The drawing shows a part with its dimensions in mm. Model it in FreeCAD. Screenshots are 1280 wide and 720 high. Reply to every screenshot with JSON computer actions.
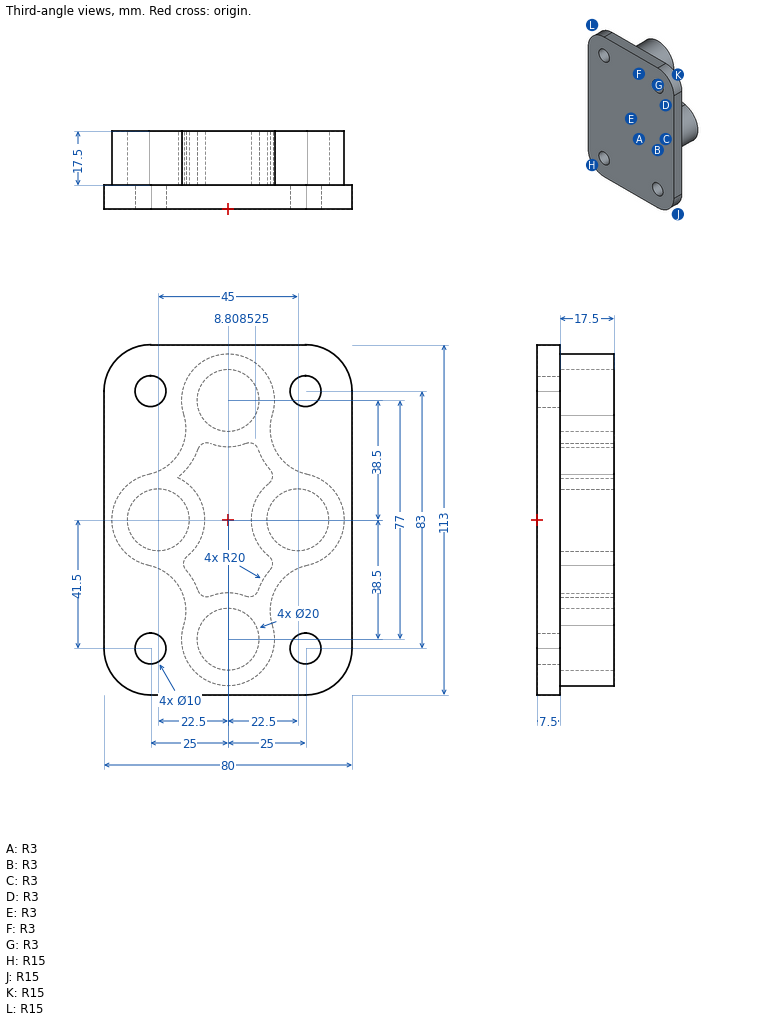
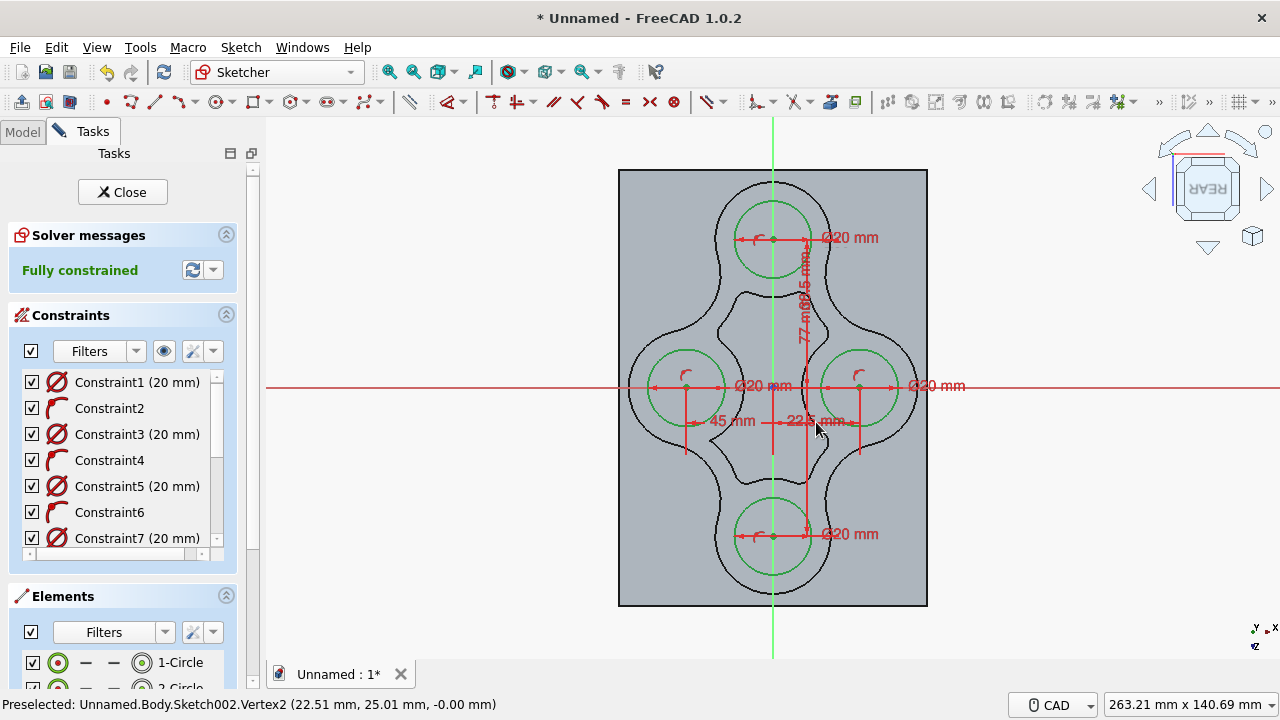
{"action": "left_click", "coordinate": [123, 192]}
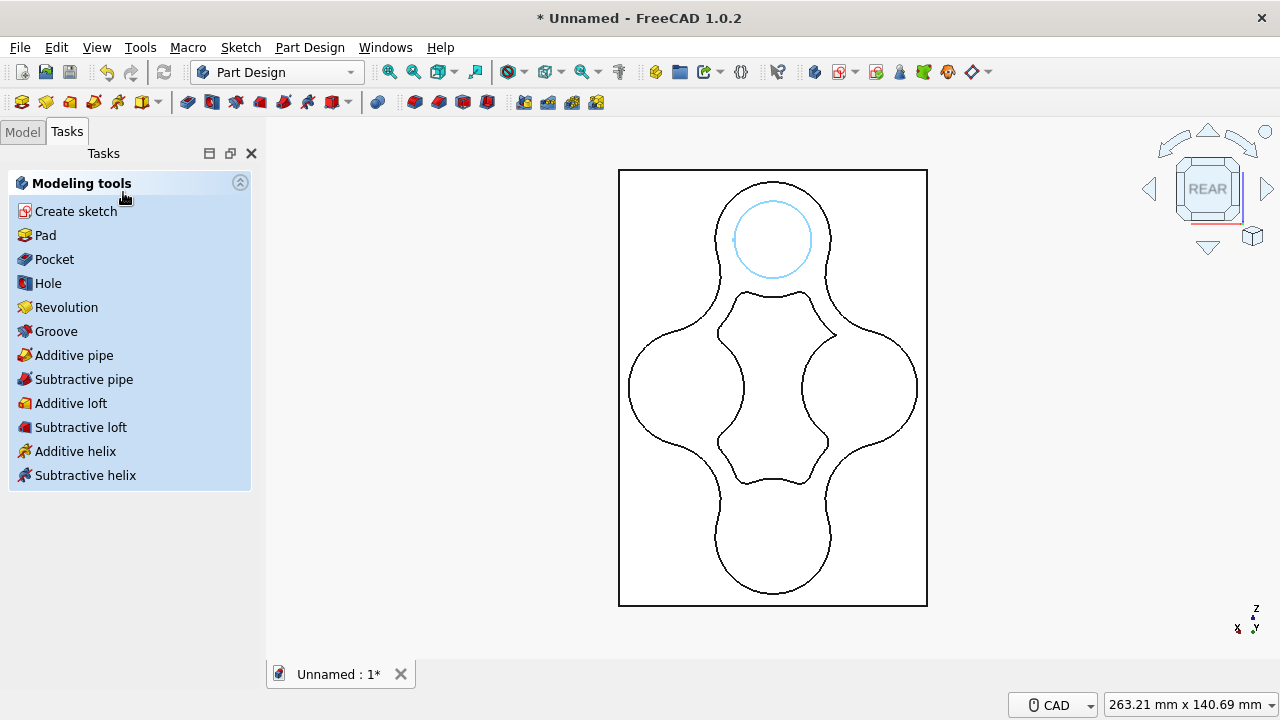
{"action": "left_click", "coordinate": [188, 102]}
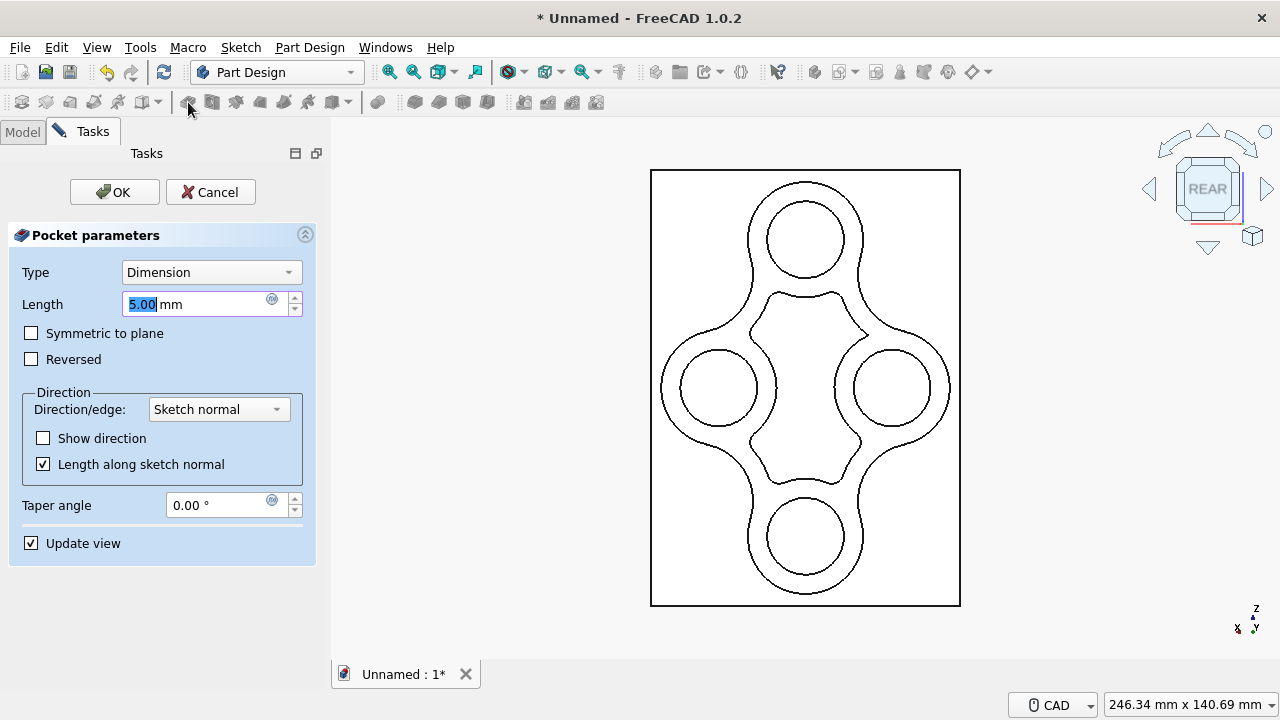
{"action": "type", "text": "17.5"}
{"action": "key", "text": "Tab"}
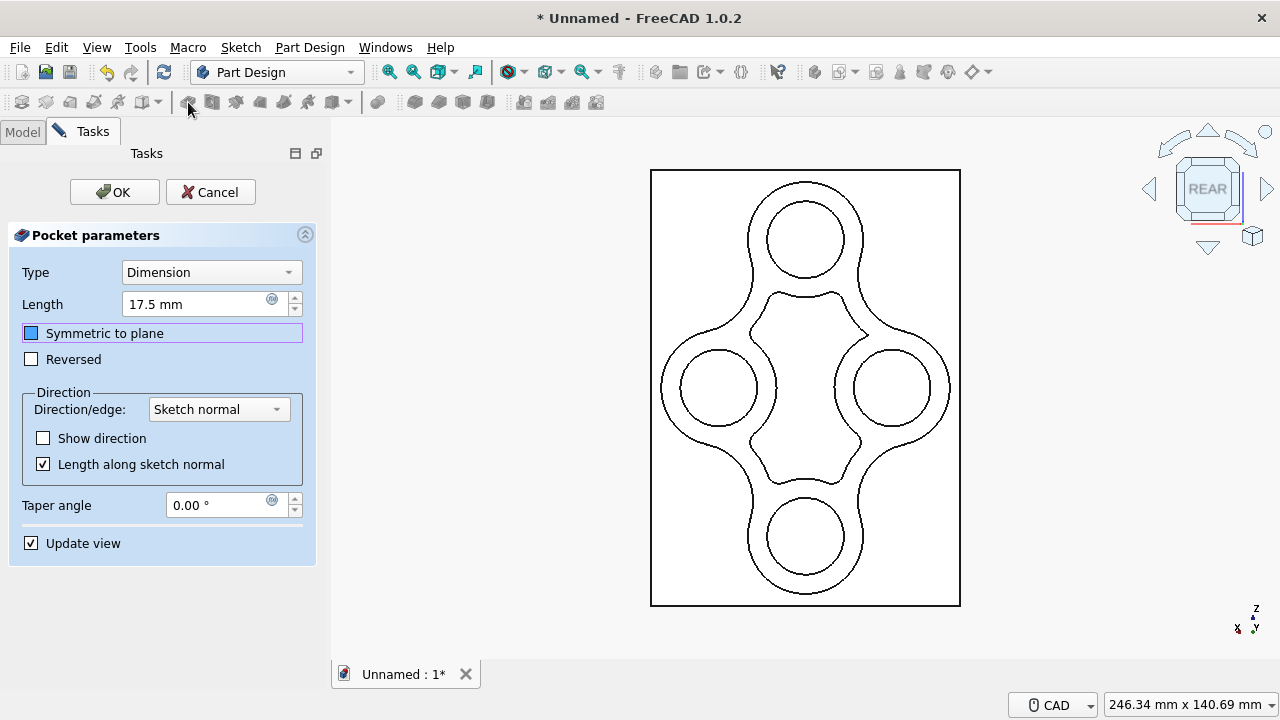
{"action": "left_click", "coordinate": [115, 192]}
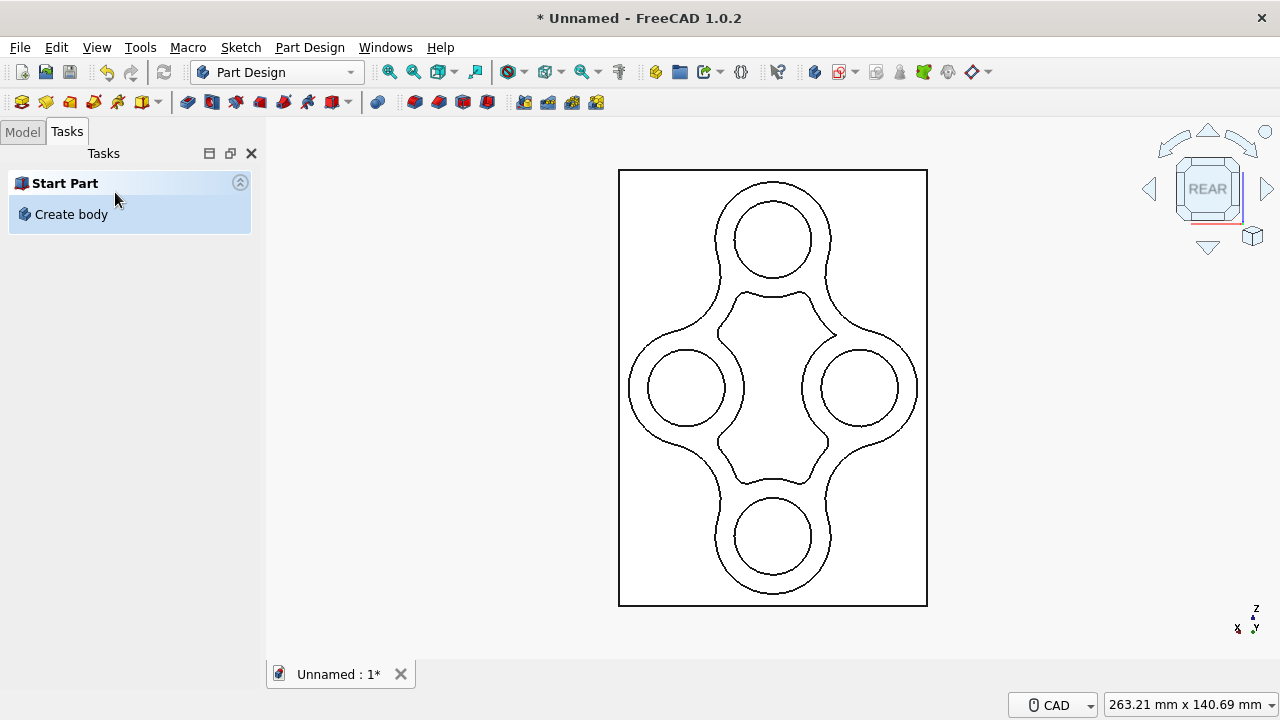
{"action": "key", "text": "0"}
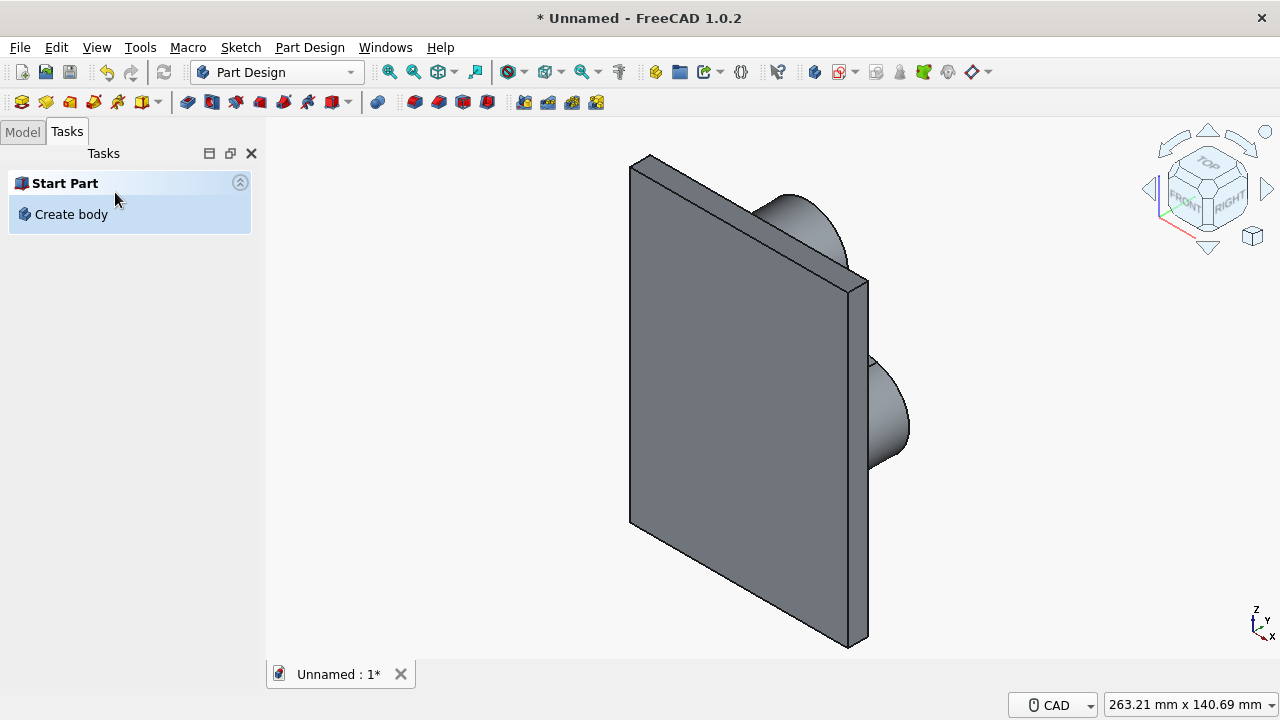
{"action": "key", "text": "2"}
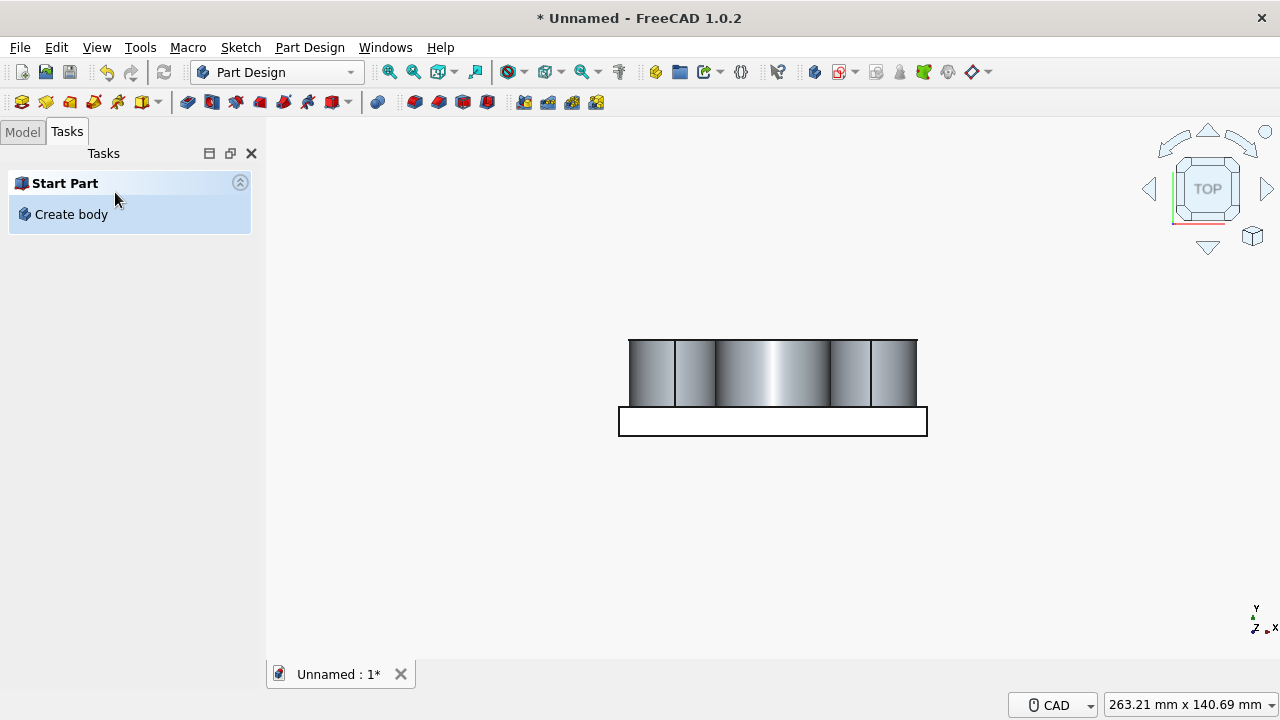
{"action": "key", "text": "v f"}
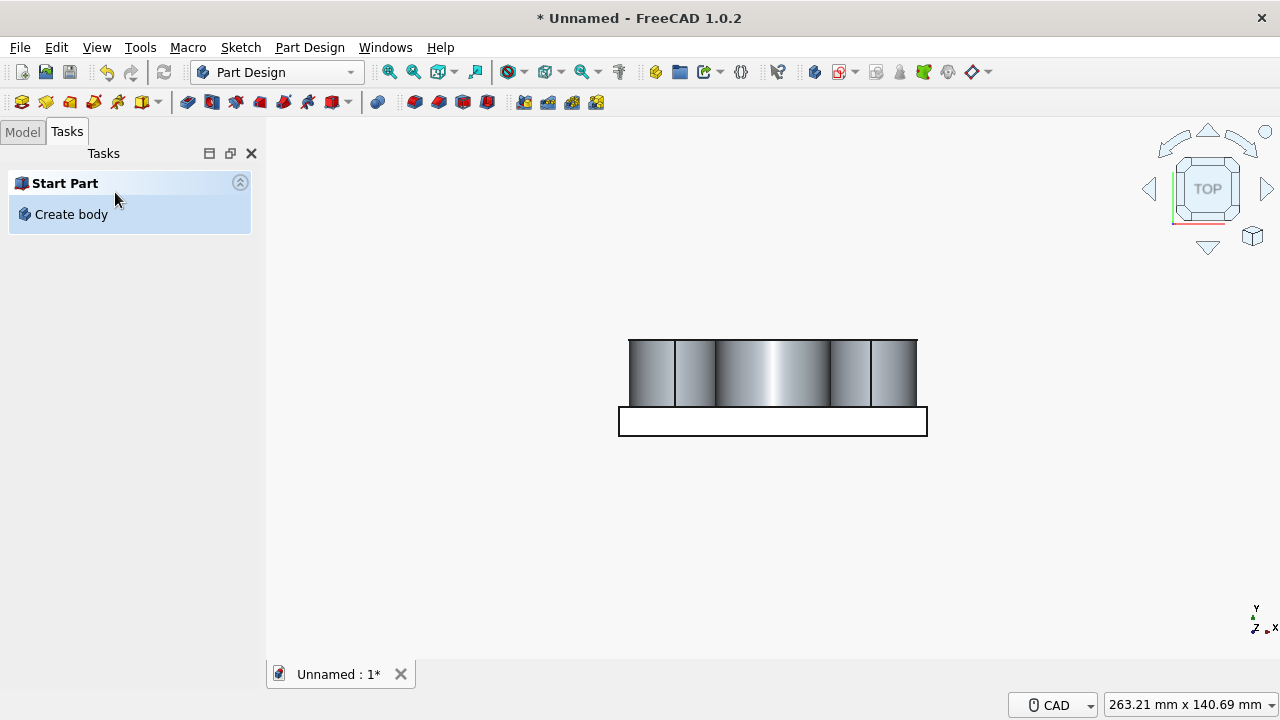
{"action": "key", "text": "1"}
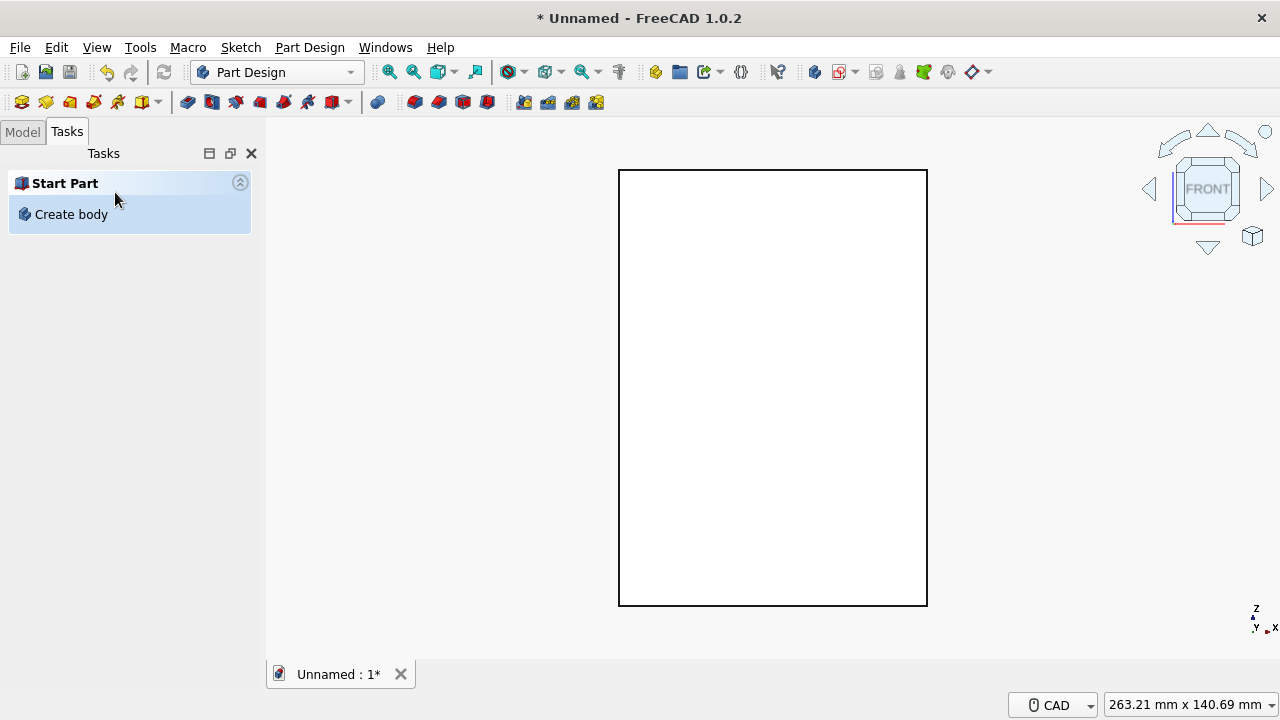
{"action": "key", "text": "3"}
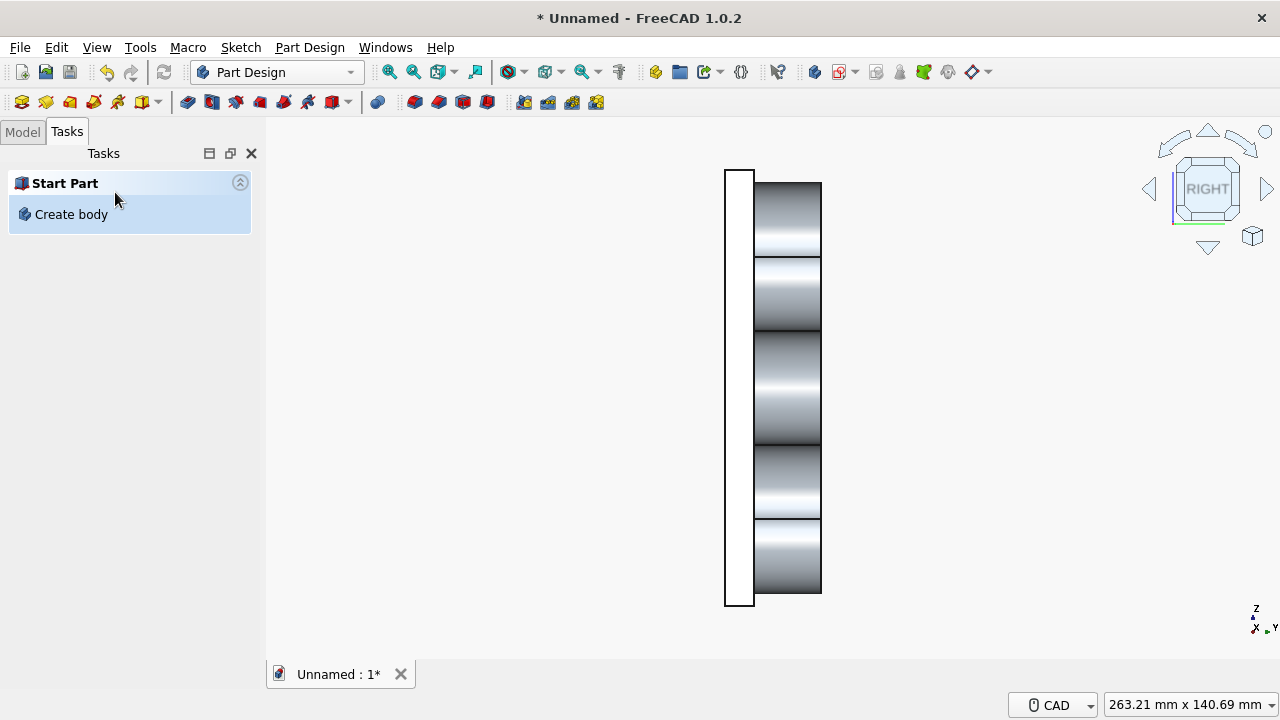
{"action": "key", "text": "5"}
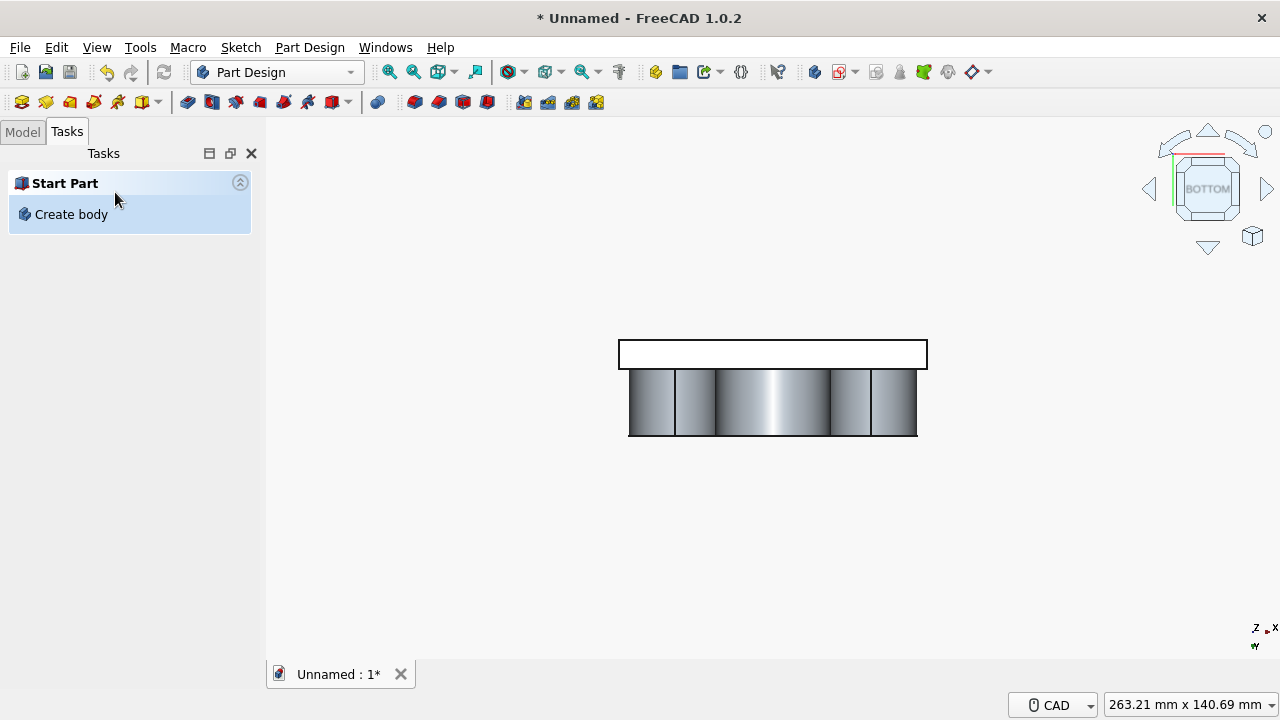
{"action": "key", "text": "v f"}